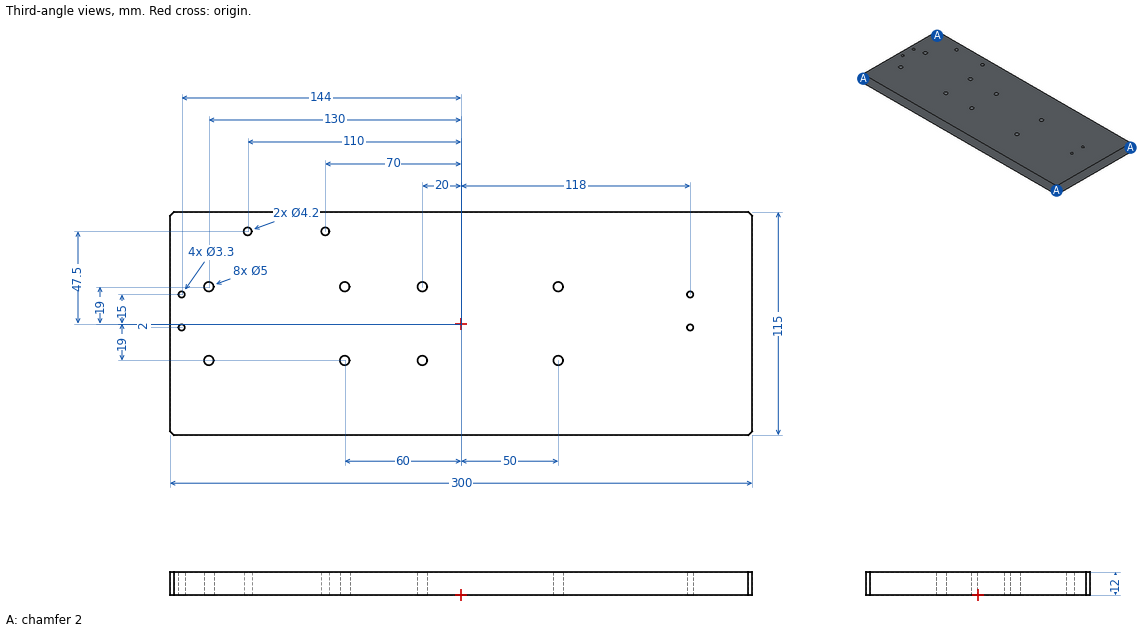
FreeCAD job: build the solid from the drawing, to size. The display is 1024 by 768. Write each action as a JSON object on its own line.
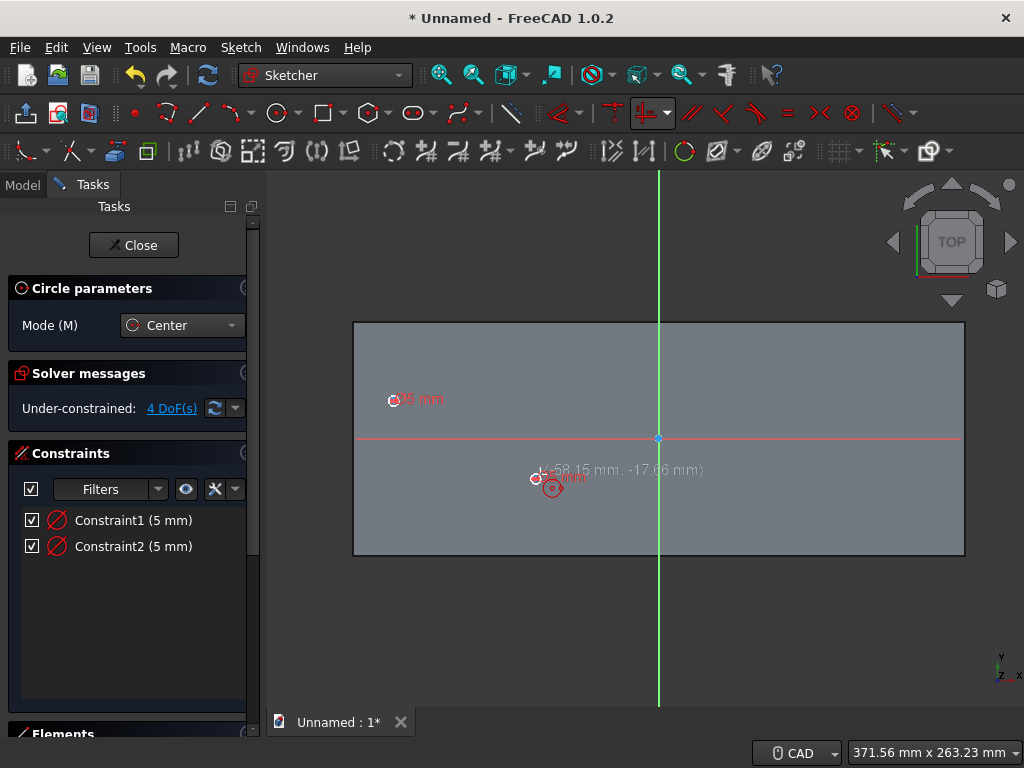
{"action": "scroll", "coordinate": [536, 400], "scroll_direction": "up", "scroll_amount": 8}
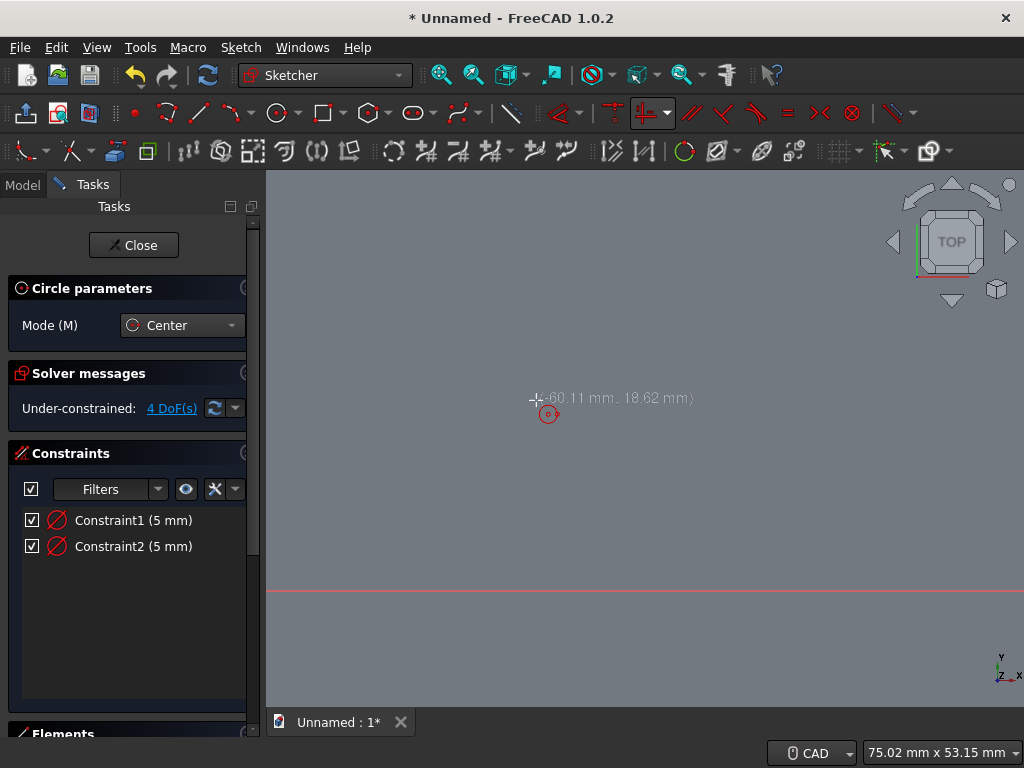
{"action": "scroll", "coordinate": [536, 400], "scroll_direction": "down", "scroll_amount": 8}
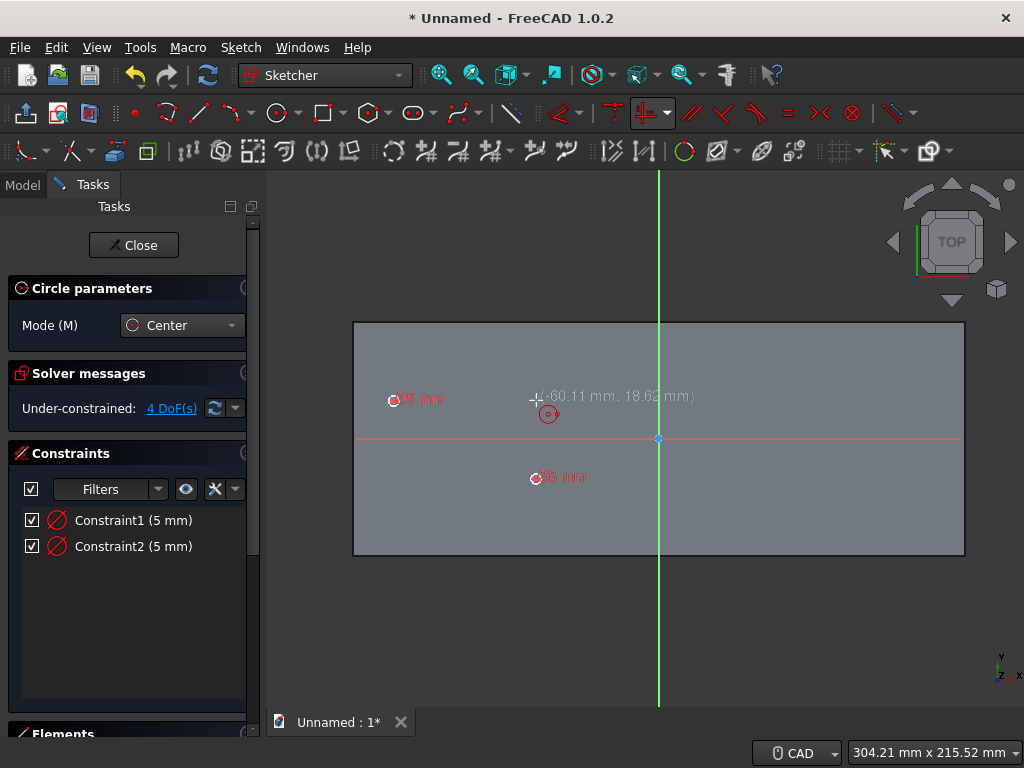
{"action": "left_click", "coordinate": [536, 400]}
{"action": "mouse_move", "coordinate": [540, 397]}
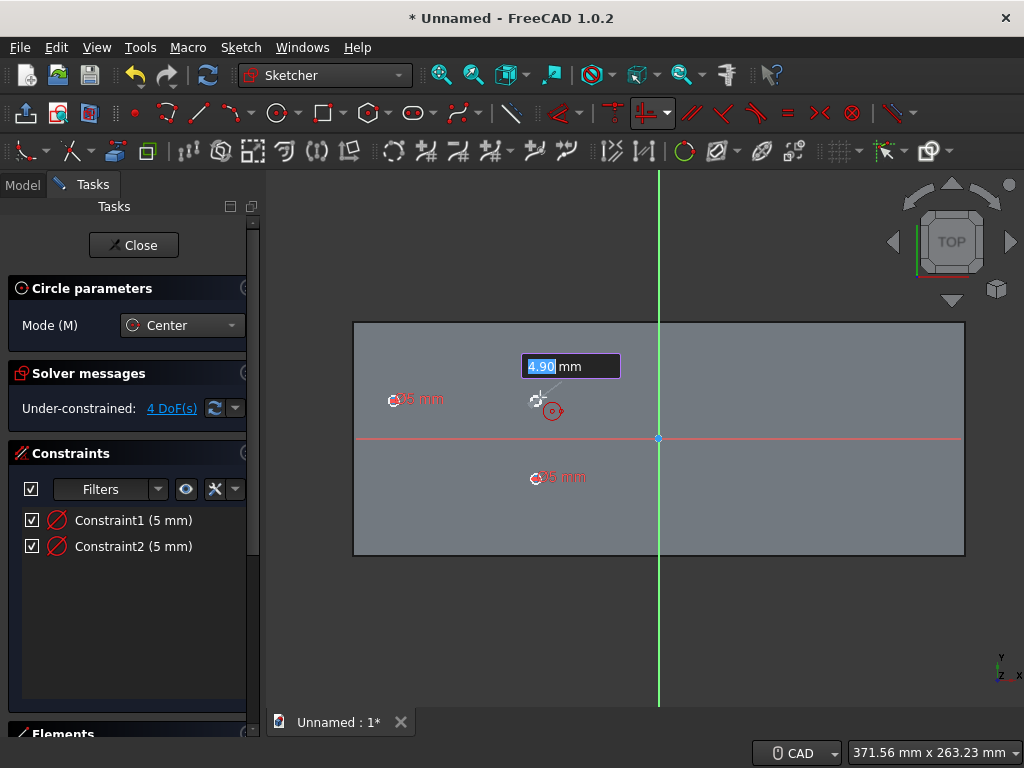
{"action": "type", "text": "5"}
{"action": "key", "text": "Return"}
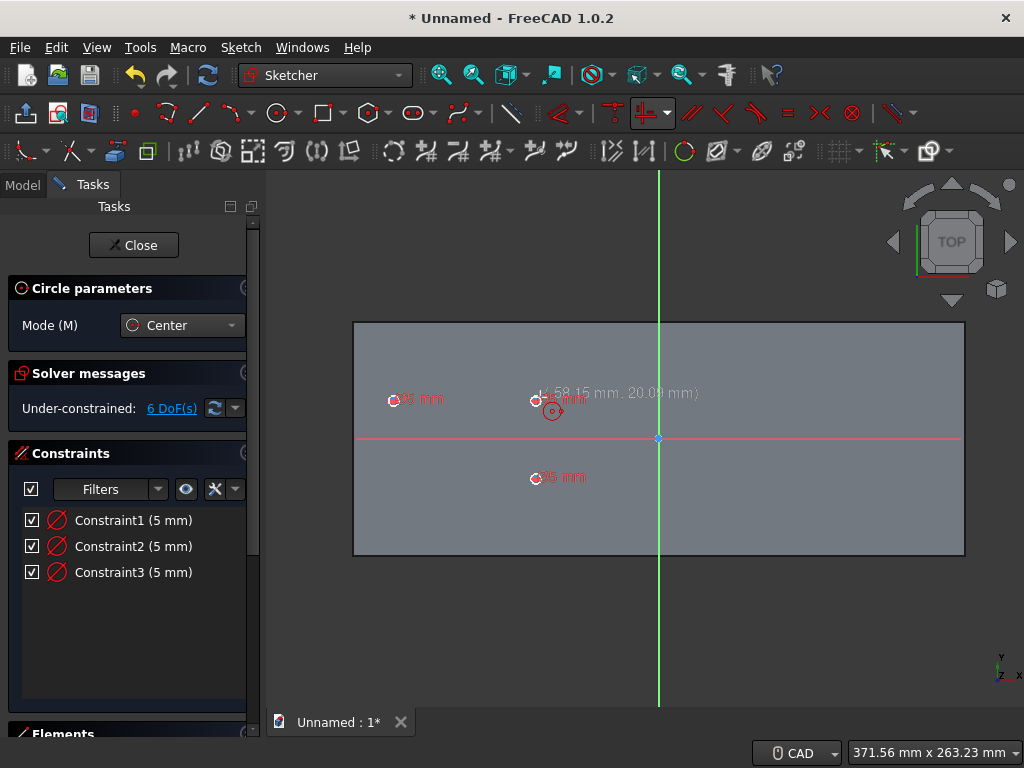
{"action": "scroll", "coordinate": [393, 478], "scroll_direction": "up", "scroll_amount": 8}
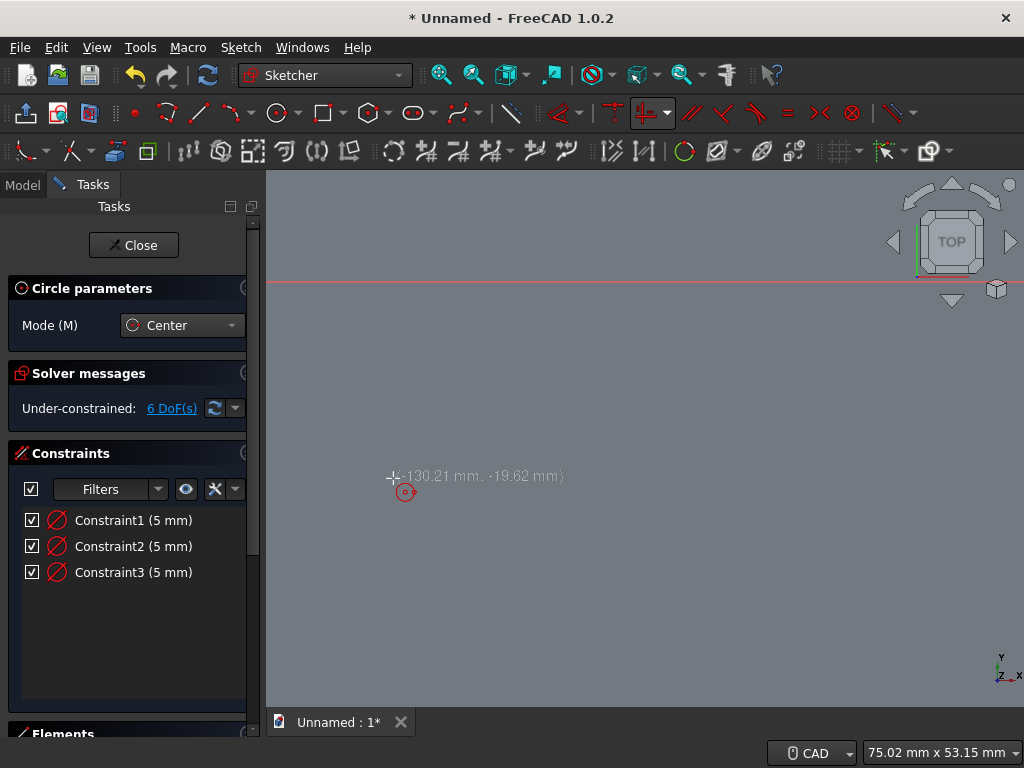
{"action": "scroll", "coordinate": [393, 478], "scroll_direction": "down", "scroll_amount": 8}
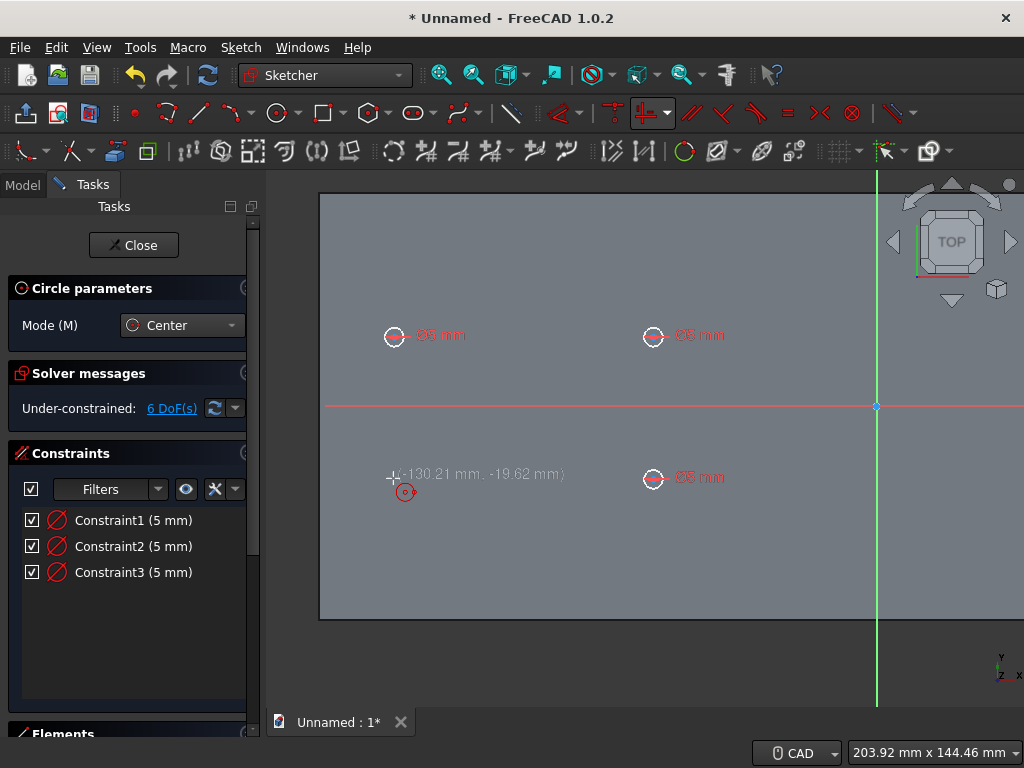
{"action": "left_click", "coordinate": [393, 478]}
{"action": "mouse_move", "coordinate": [397, 474]}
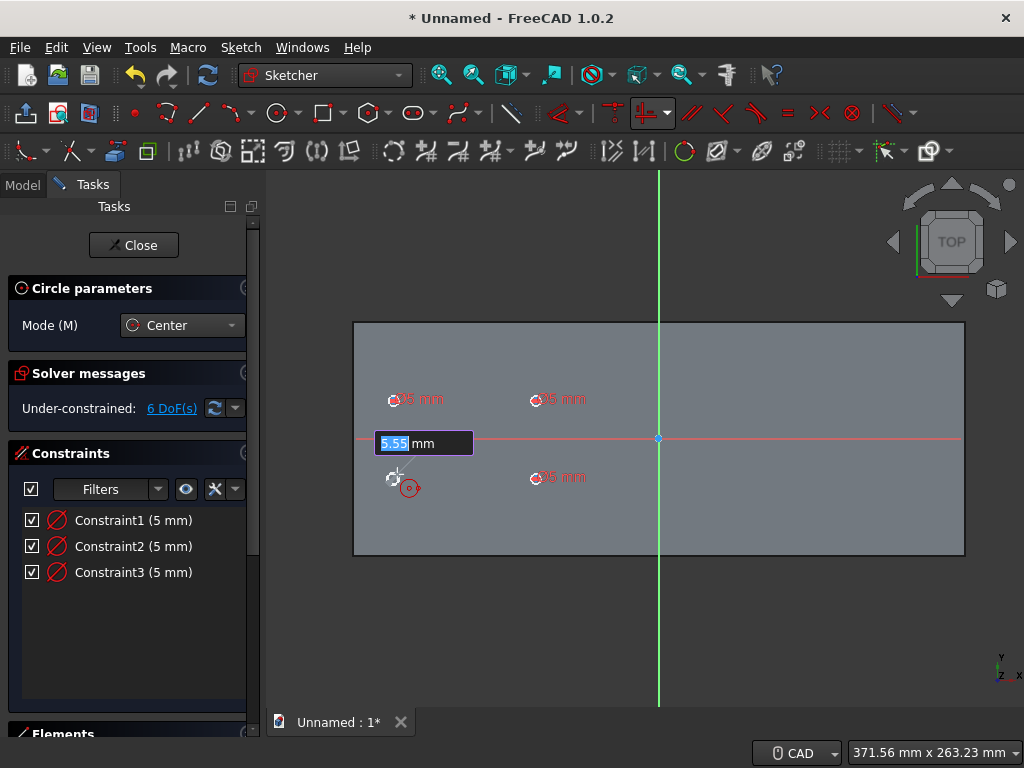
{"action": "type", "text": "5"}
{"action": "key", "text": "Return"}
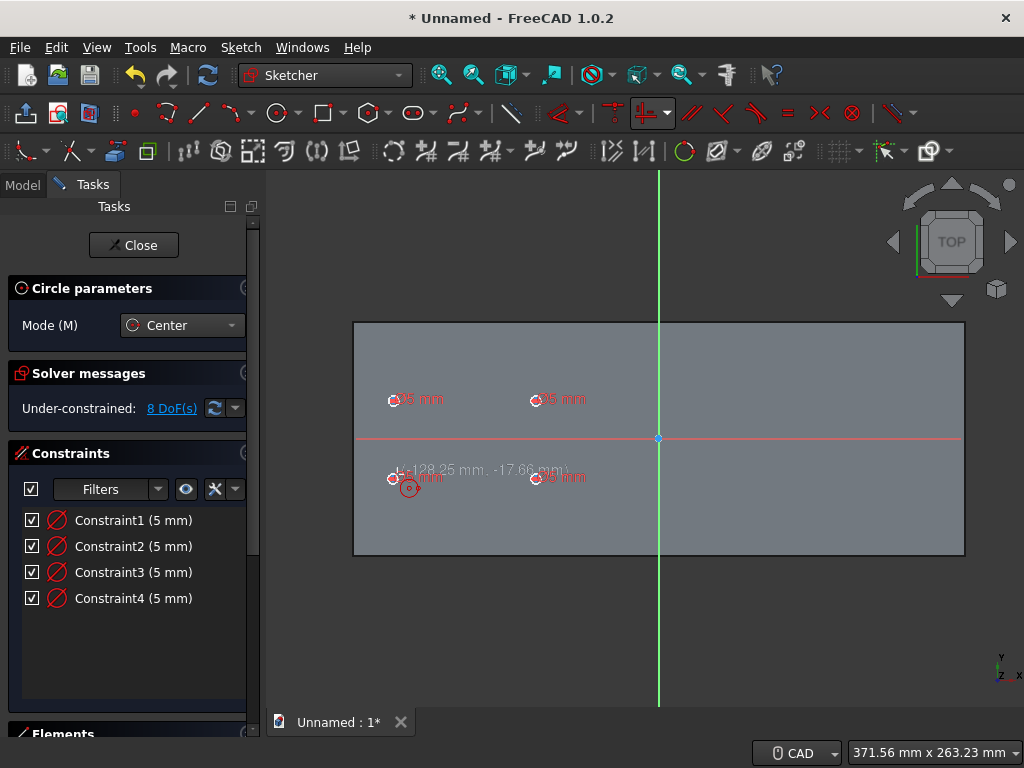
{"action": "scroll", "coordinate": [618, 400], "scroll_direction": "up", "scroll_amount": 8}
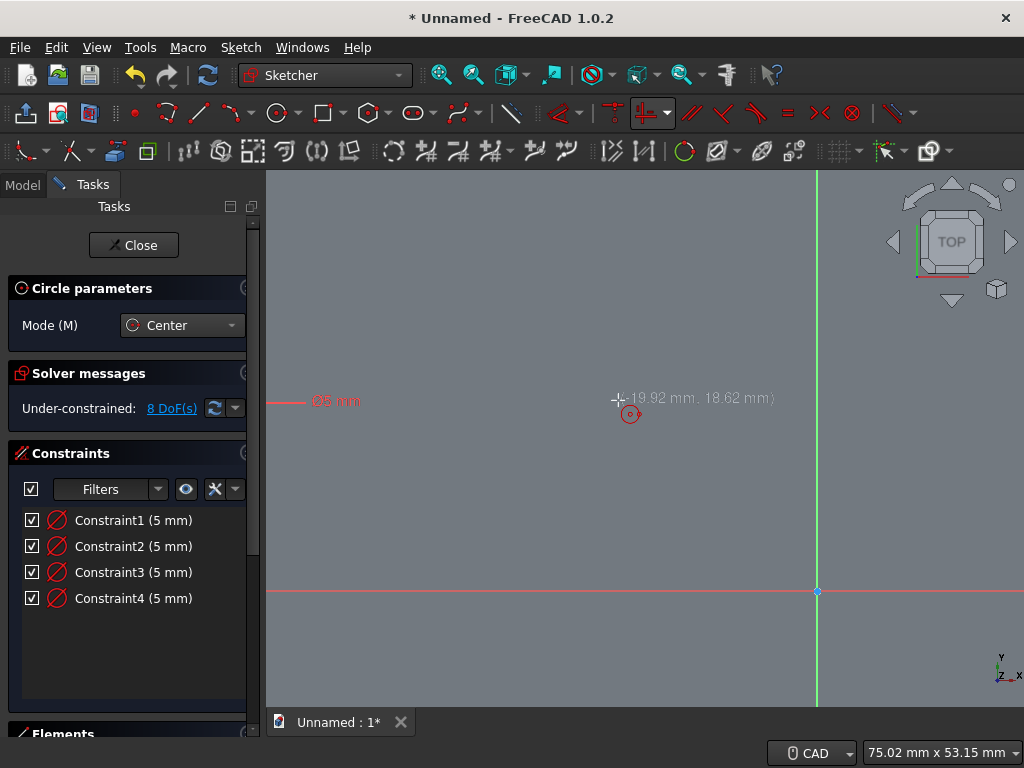
{"action": "scroll", "coordinate": [618, 400], "scroll_direction": "down", "scroll_amount": 8}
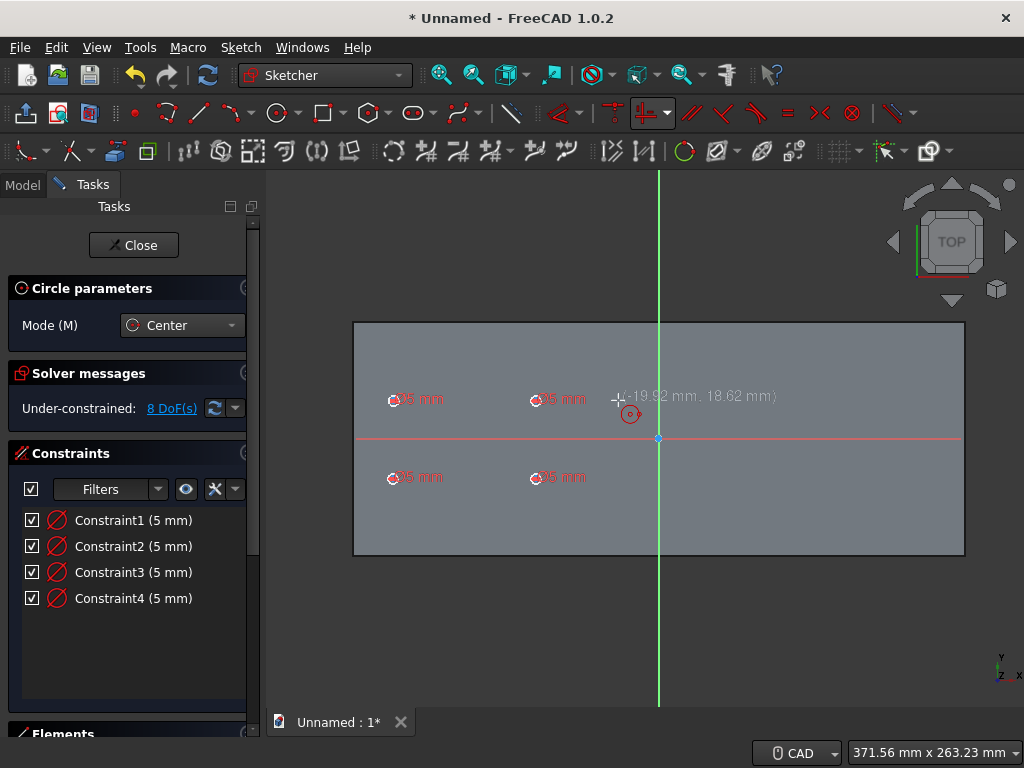
{"action": "left_click", "coordinate": [618, 400]}
{"action": "mouse_move", "coordinate": [621, 397]}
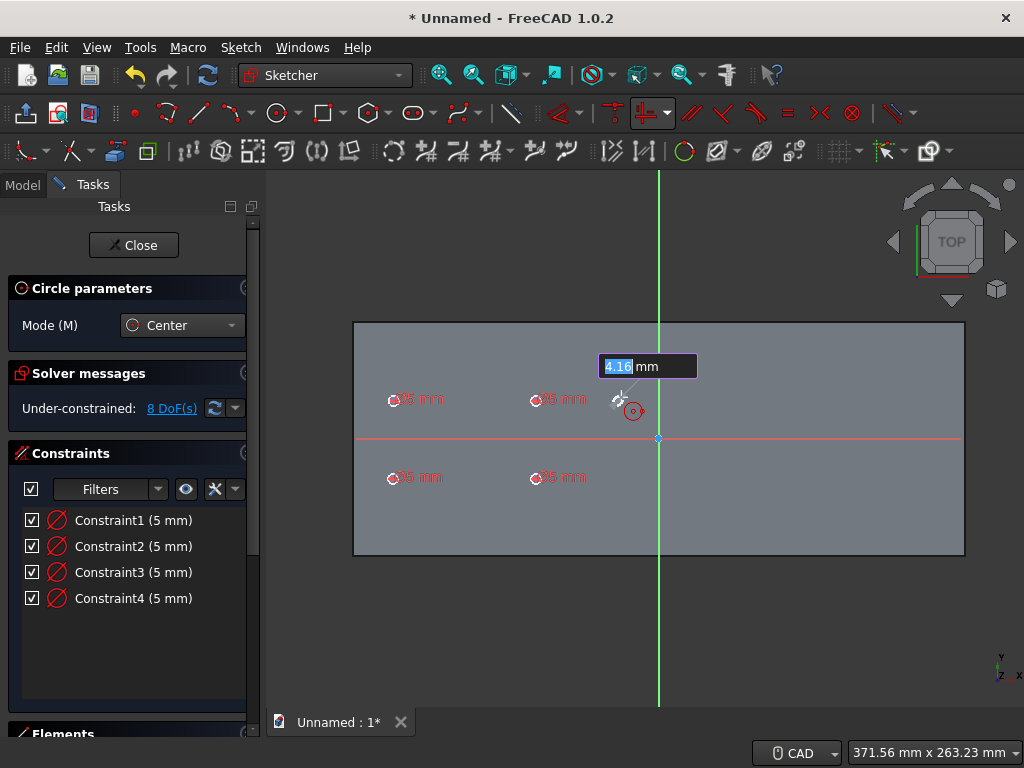
{"action": "type", "text": "5"}
{"action": "key", "text": "Return"}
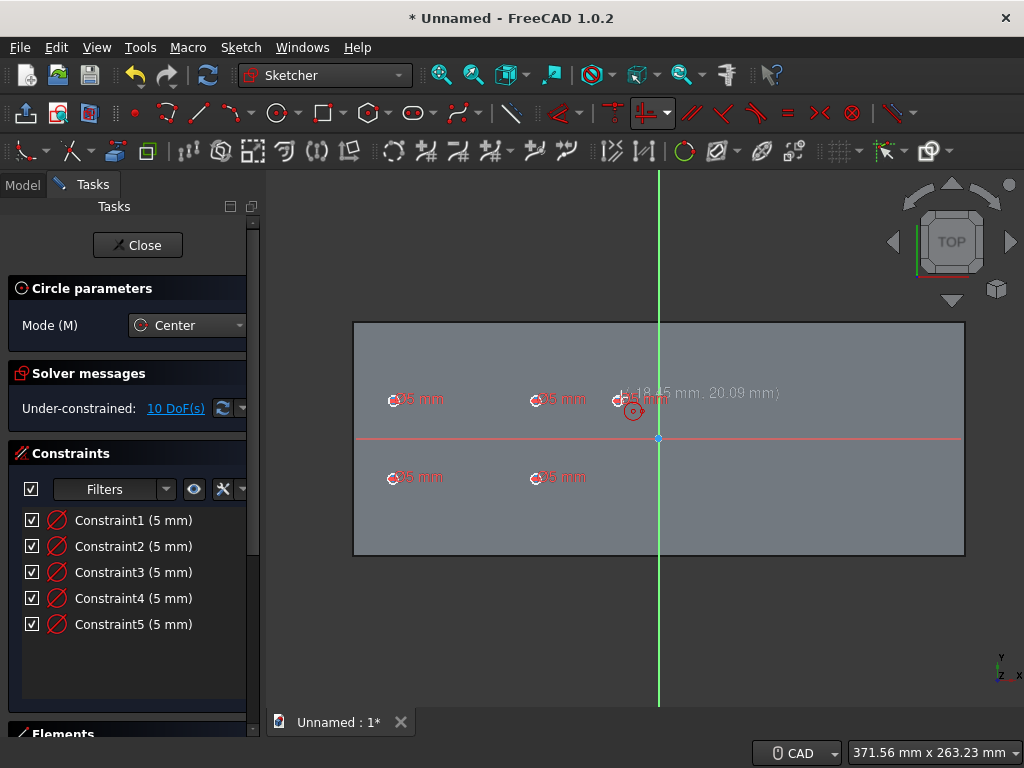
{"action": "scroll", "coordinate": [761, 478], "scroll_direction": "up", "scroll_amount": 8}